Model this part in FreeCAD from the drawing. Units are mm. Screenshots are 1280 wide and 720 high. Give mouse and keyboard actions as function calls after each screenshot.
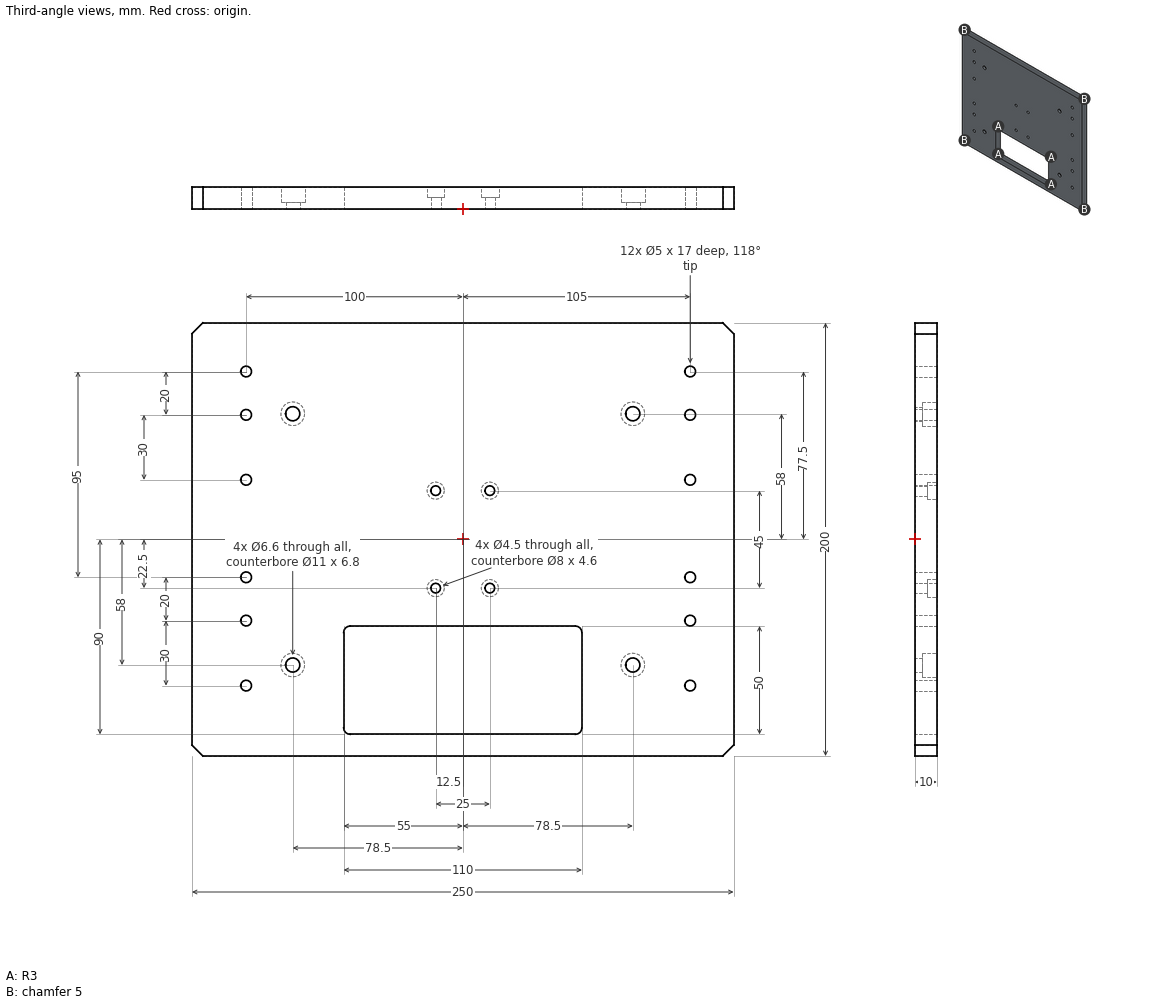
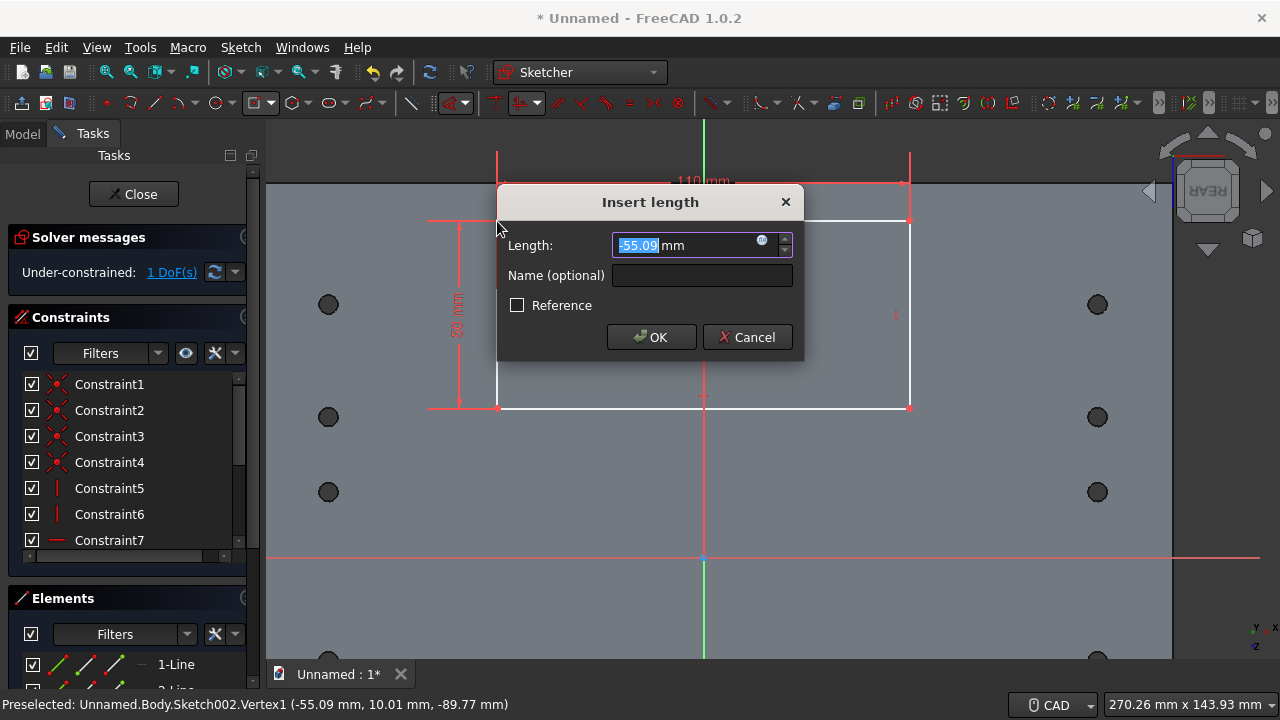
text(-55)
key(Return)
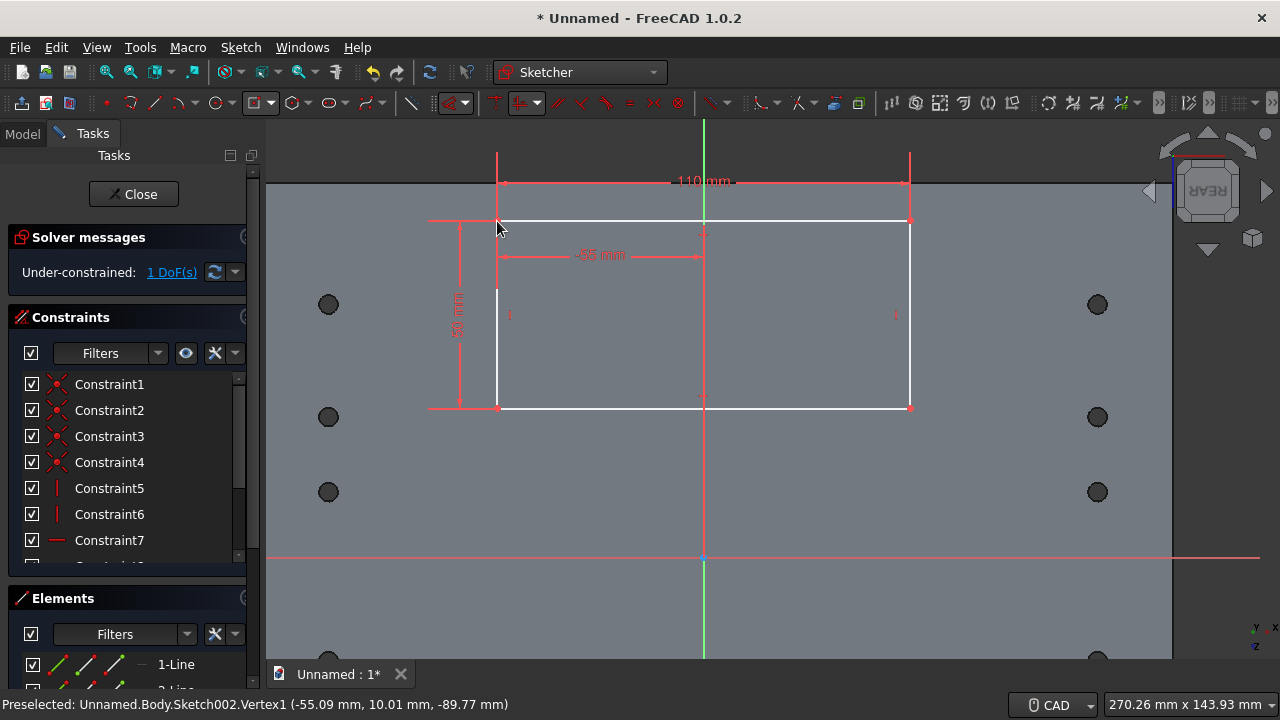
click(497, 221)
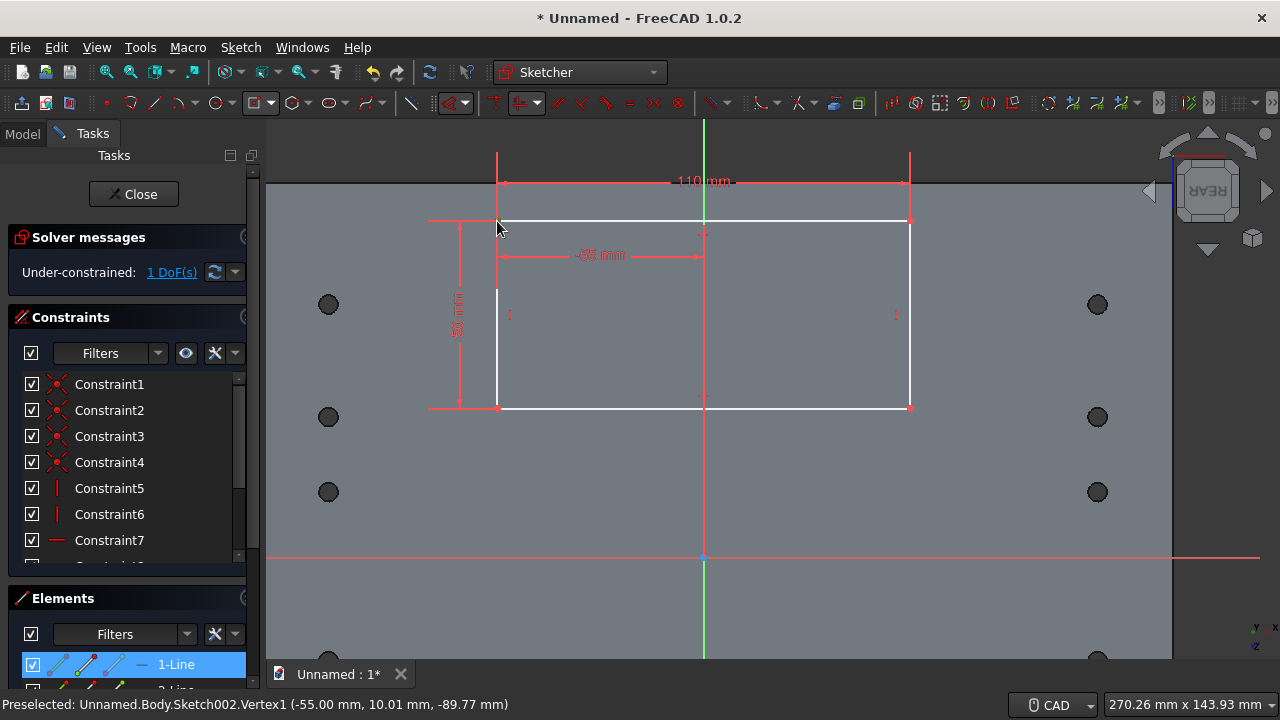
click(468, 104)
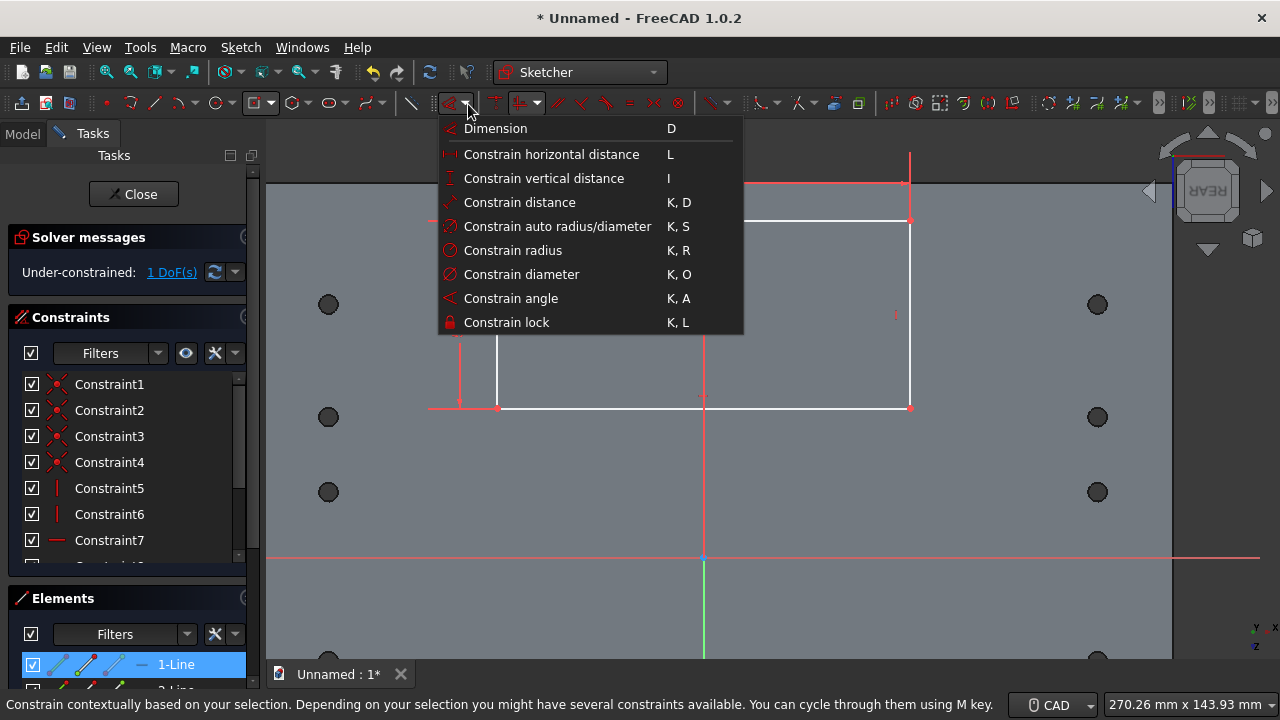
click(591, 178)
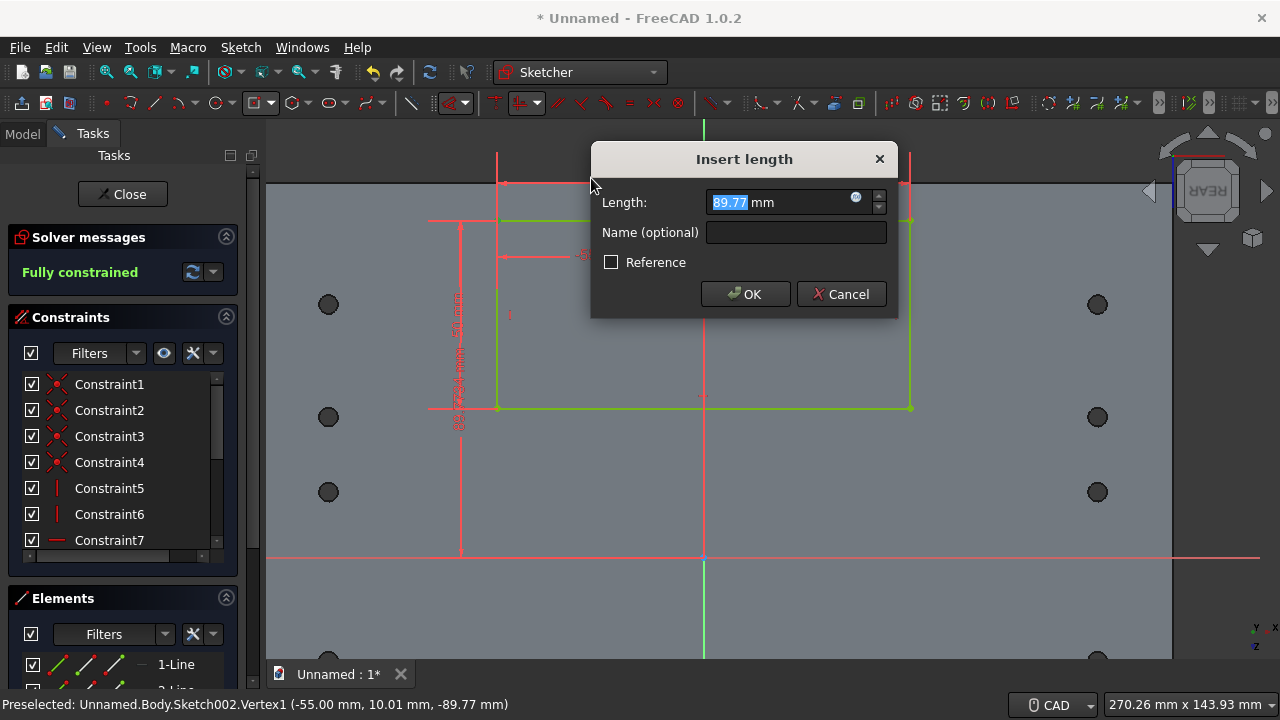
text(90)
key(Return)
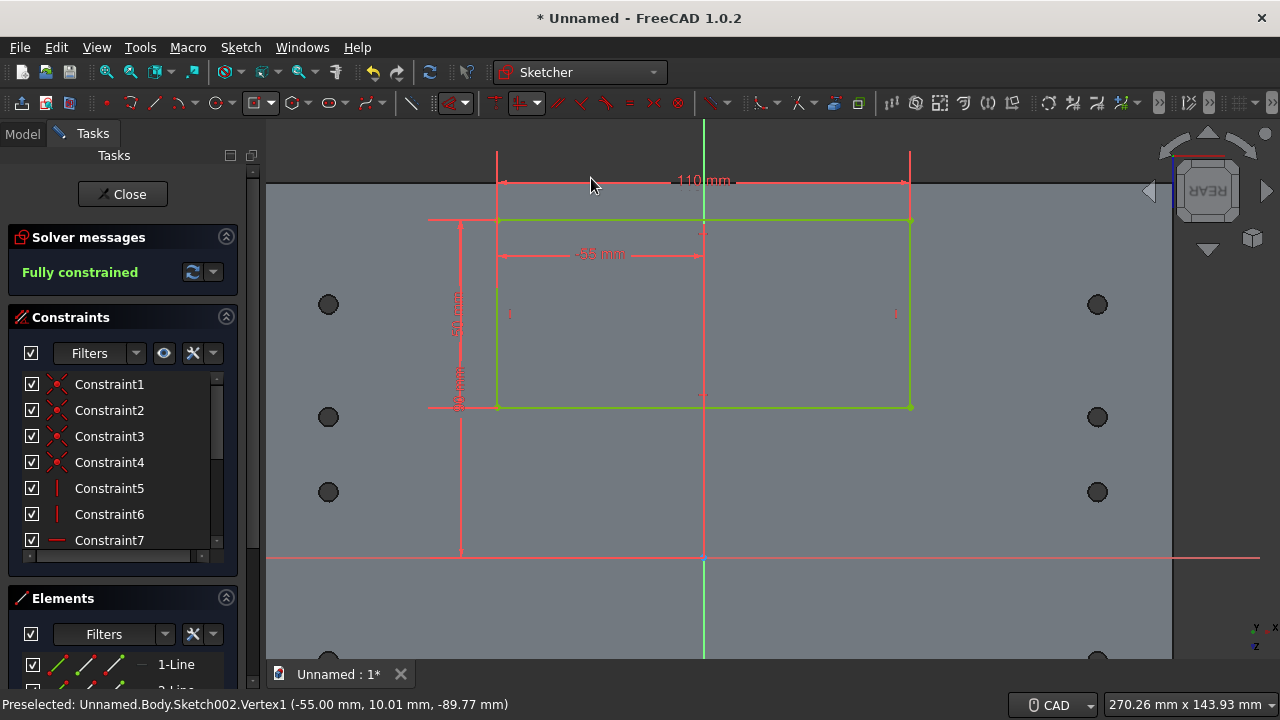
click(123, 194)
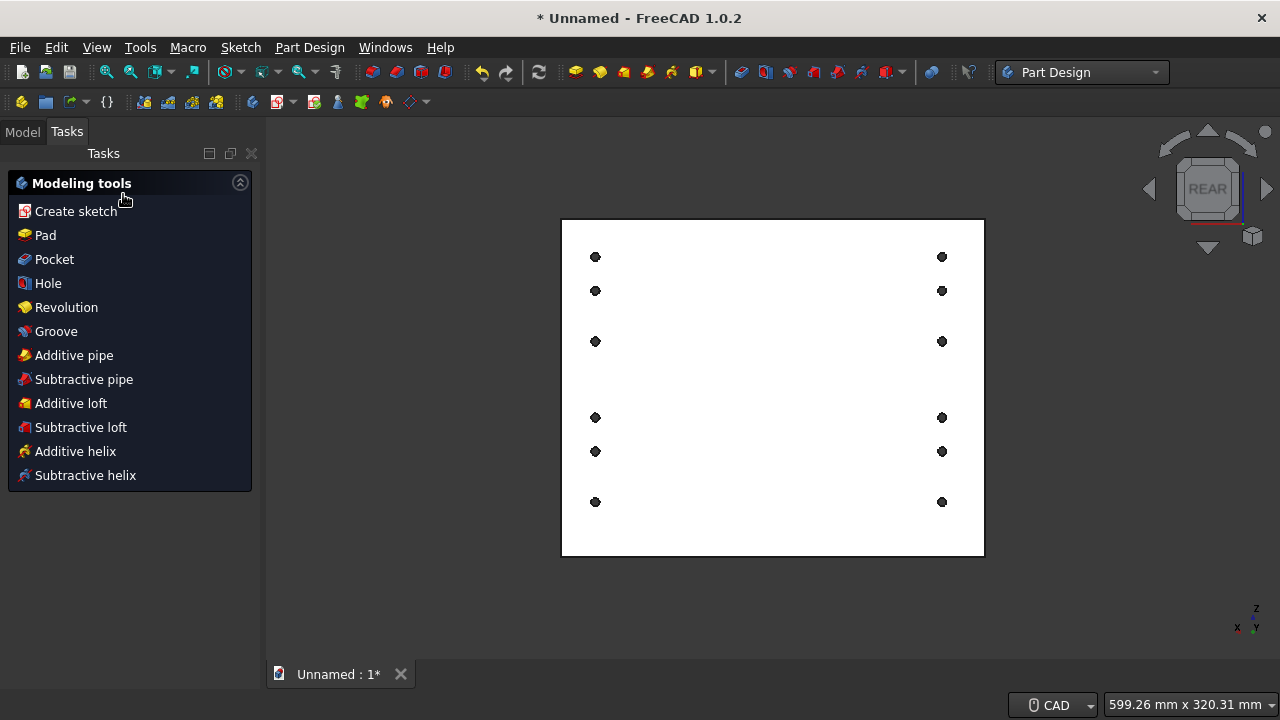
click(742, 72)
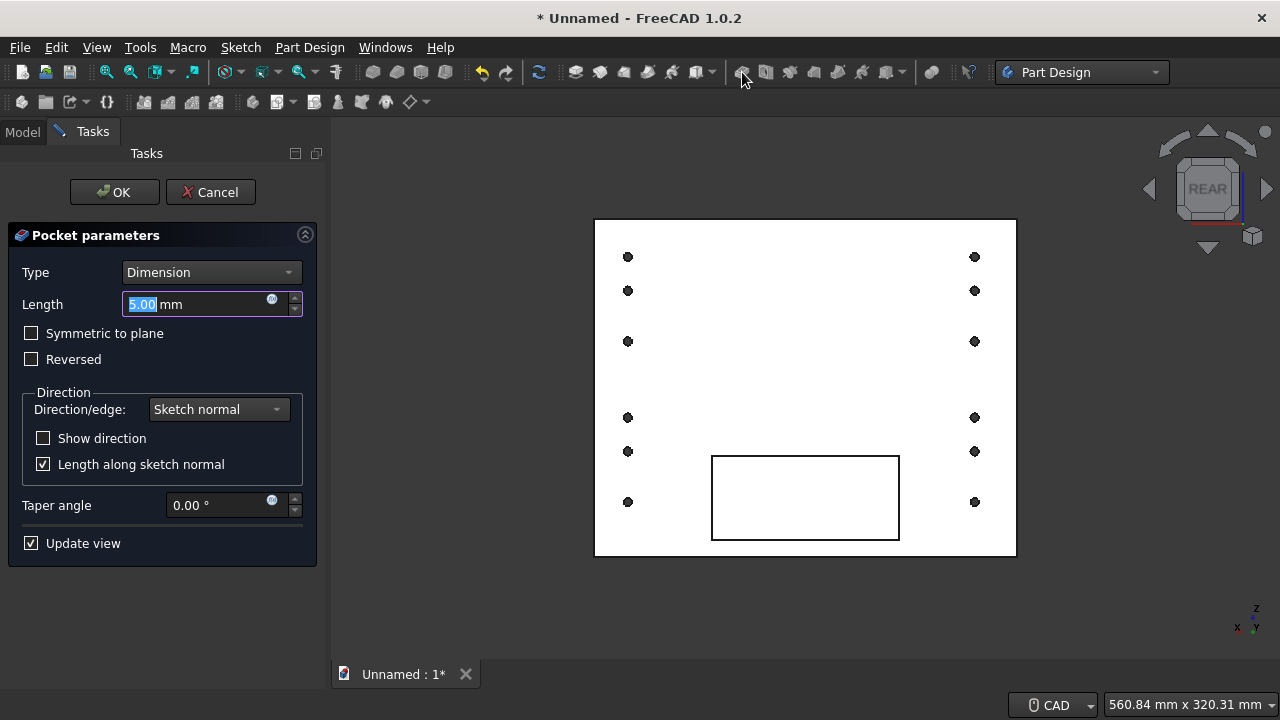
click(212, 272)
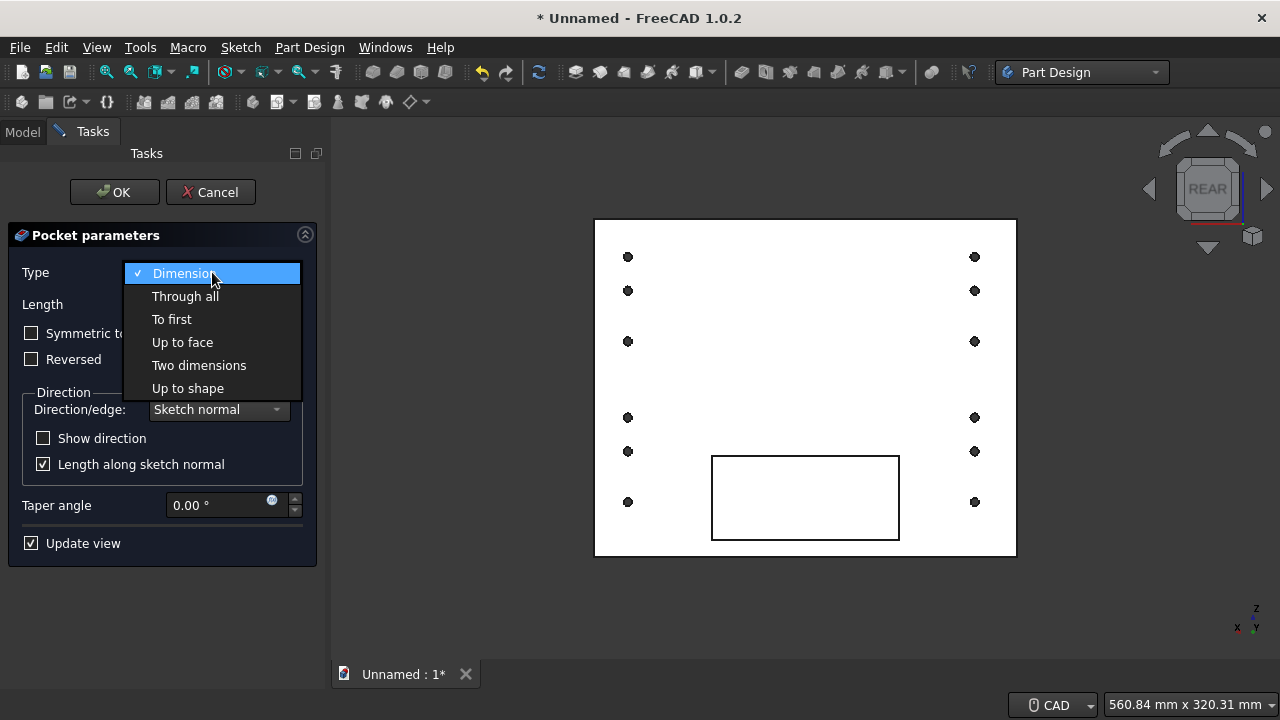
click(212, 296)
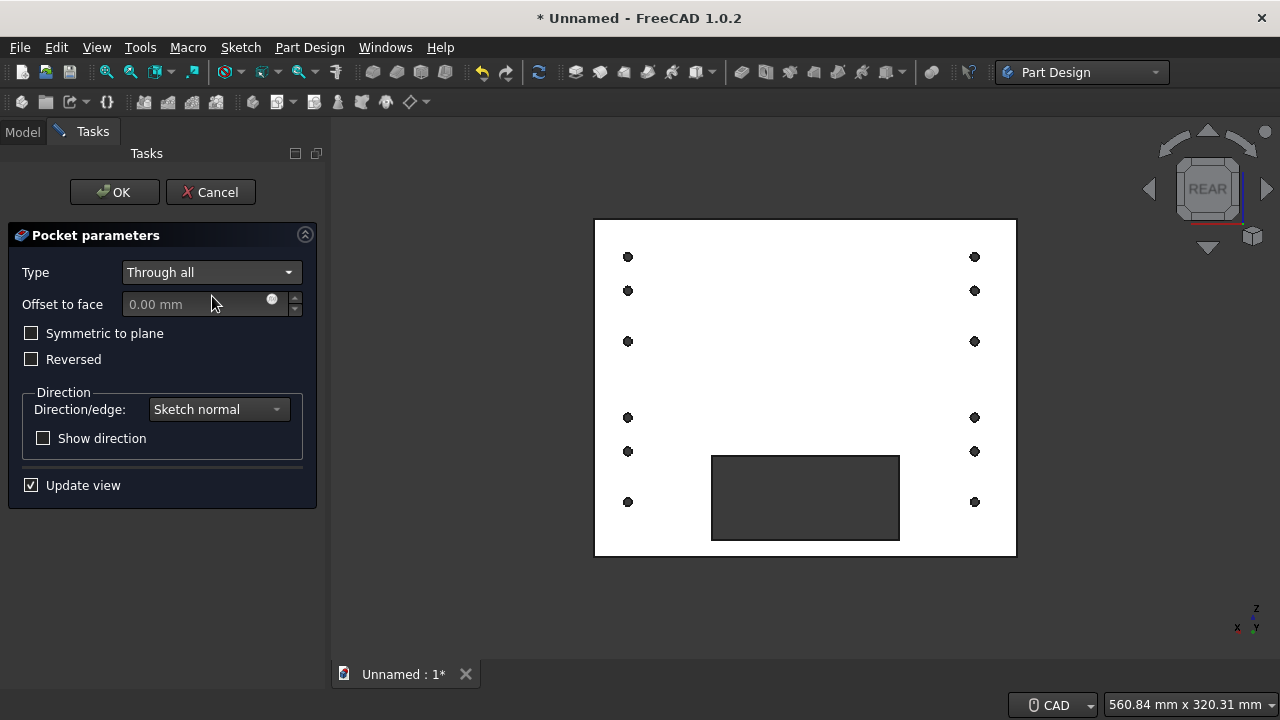
click(115, 192)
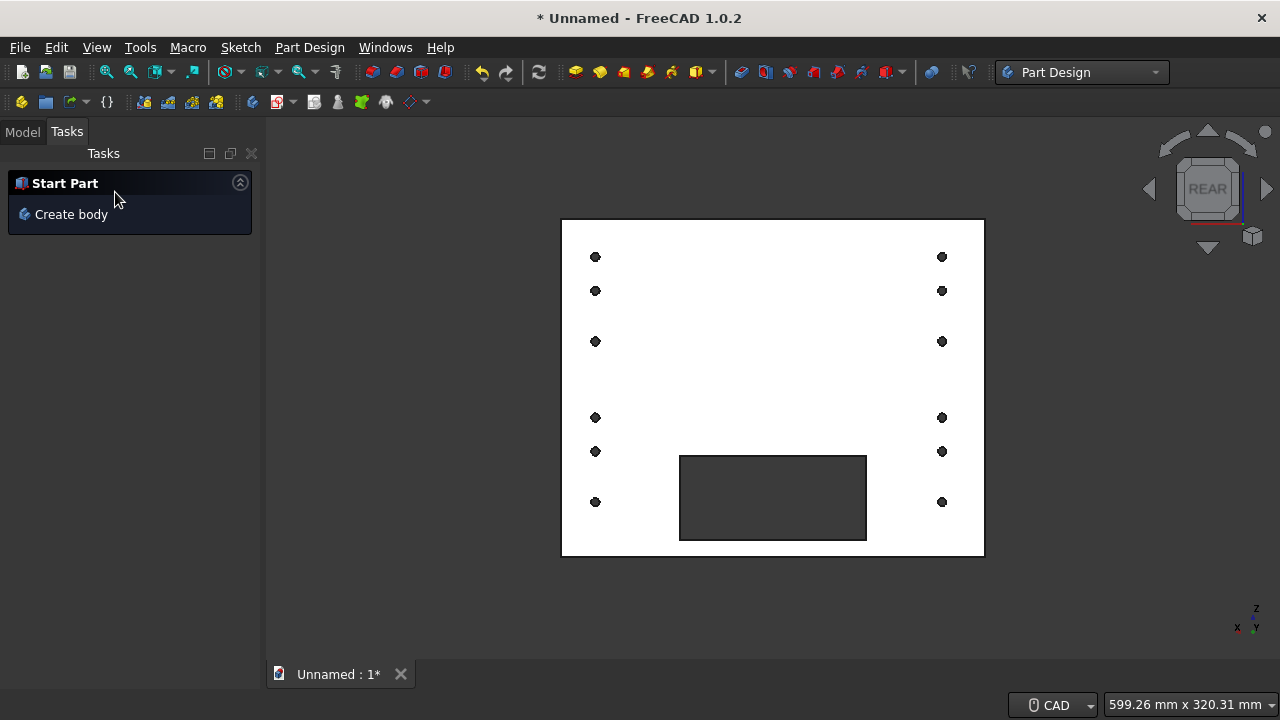
scroll(866, 455, up, 5)